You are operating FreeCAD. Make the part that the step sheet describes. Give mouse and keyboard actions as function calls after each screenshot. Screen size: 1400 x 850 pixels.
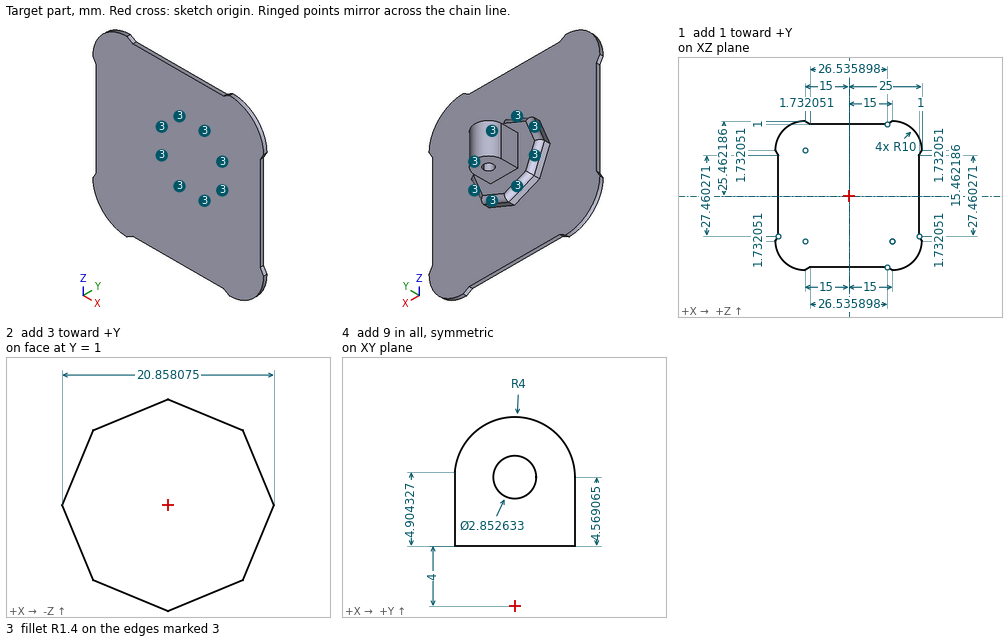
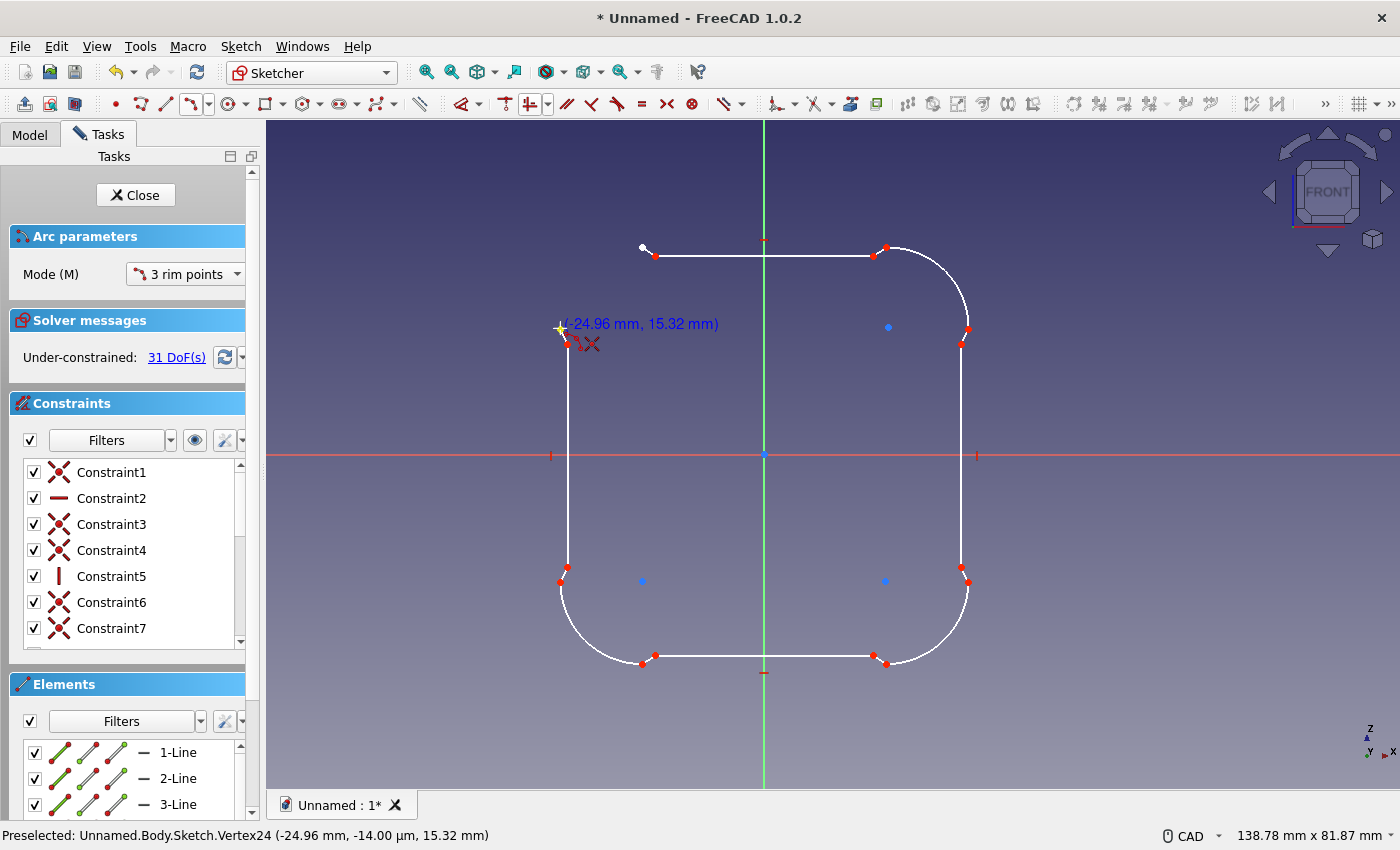
scroll(642, 247, up, 4)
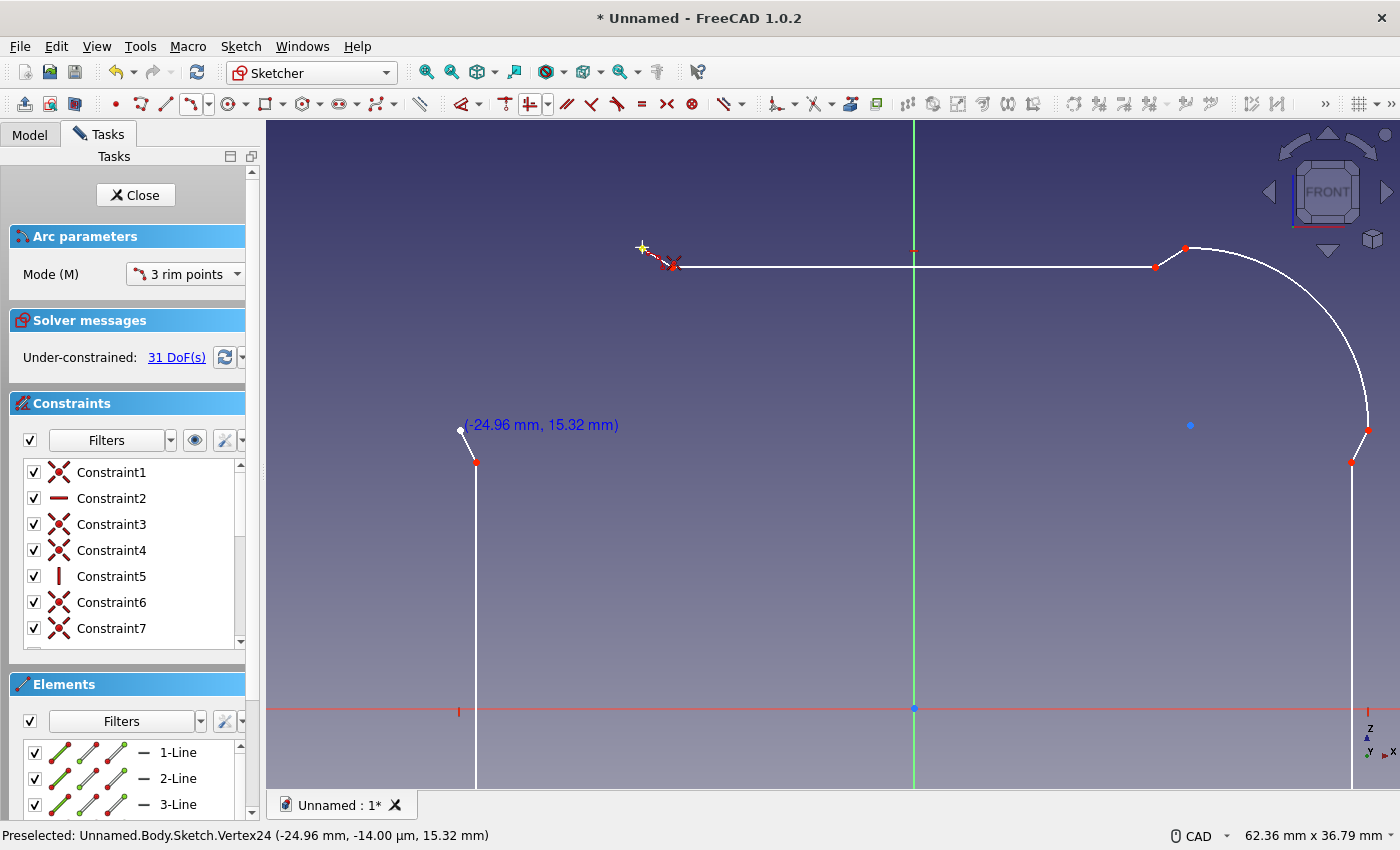
click(642, 248)
click(513, 299)
key(Escape)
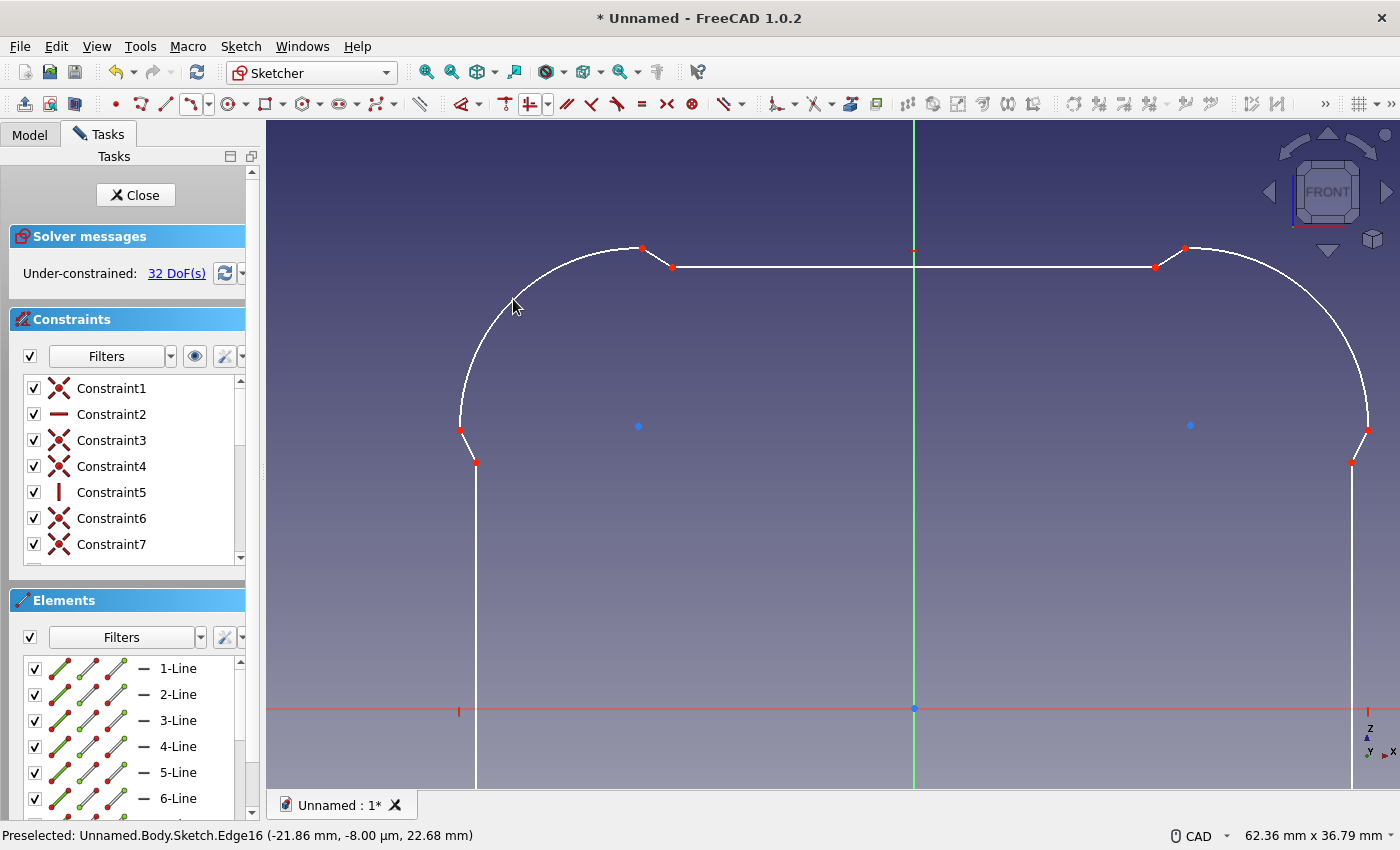
scroll(642, 247, down, 4)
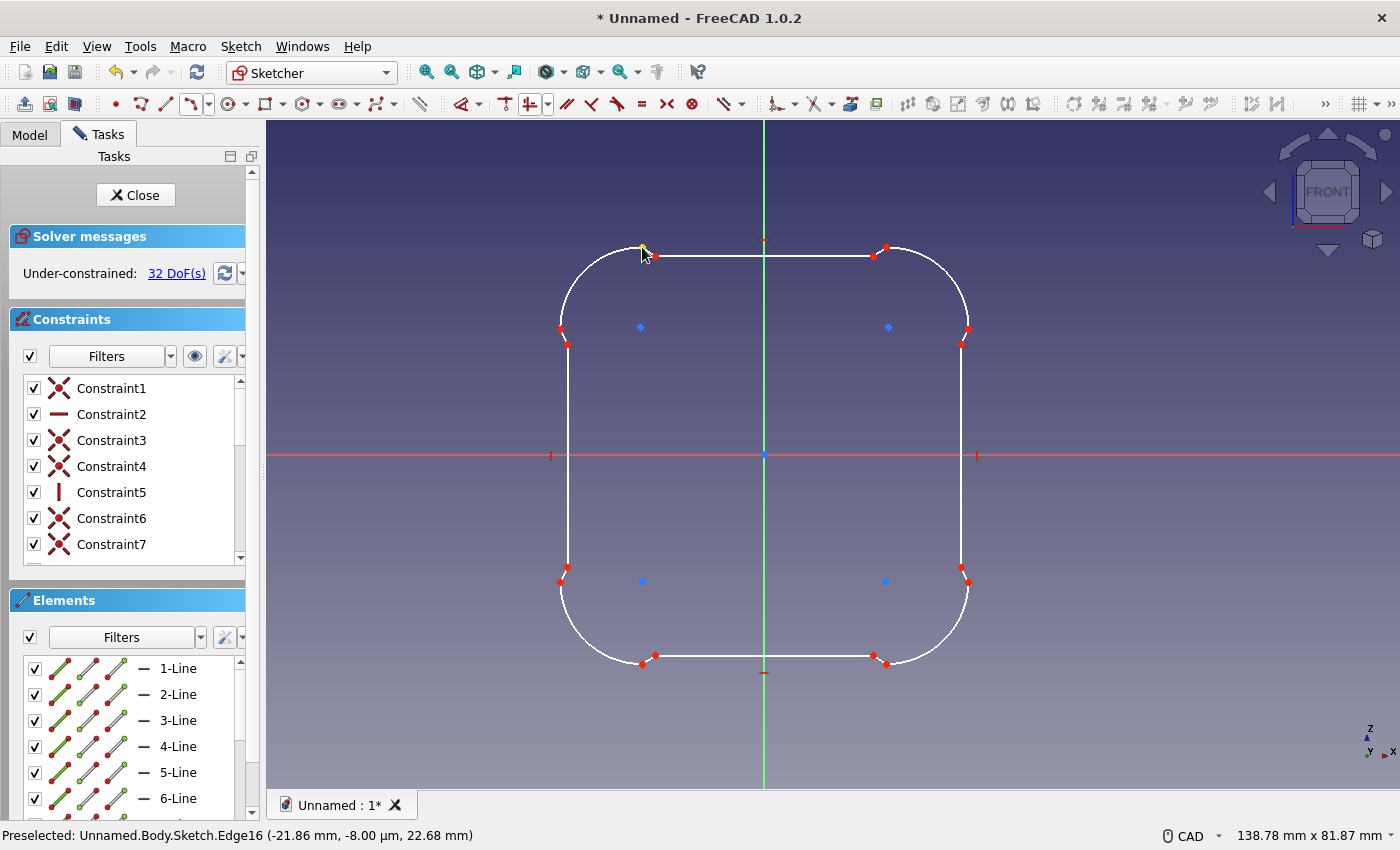
click(960, 292)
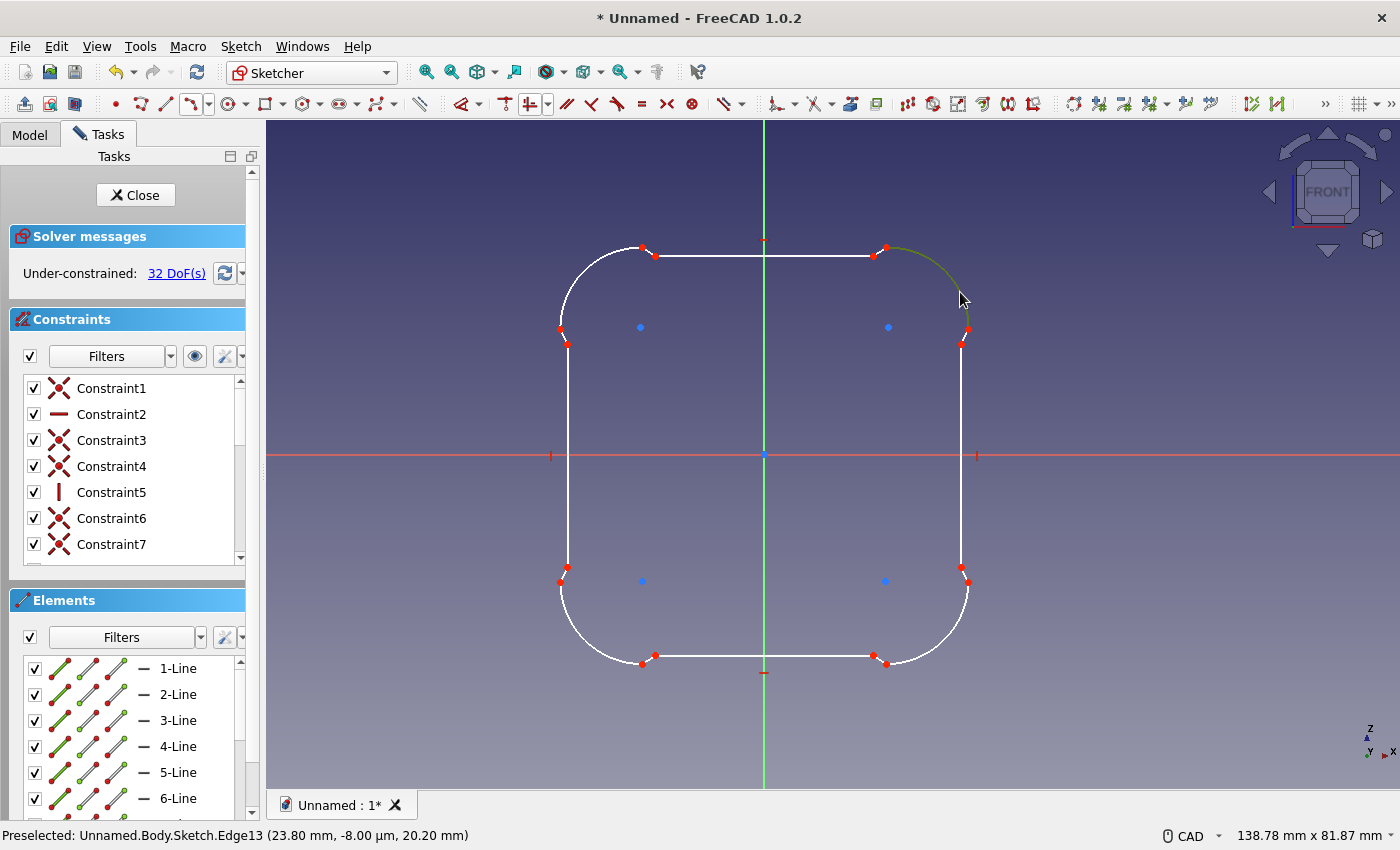
click(924, 655)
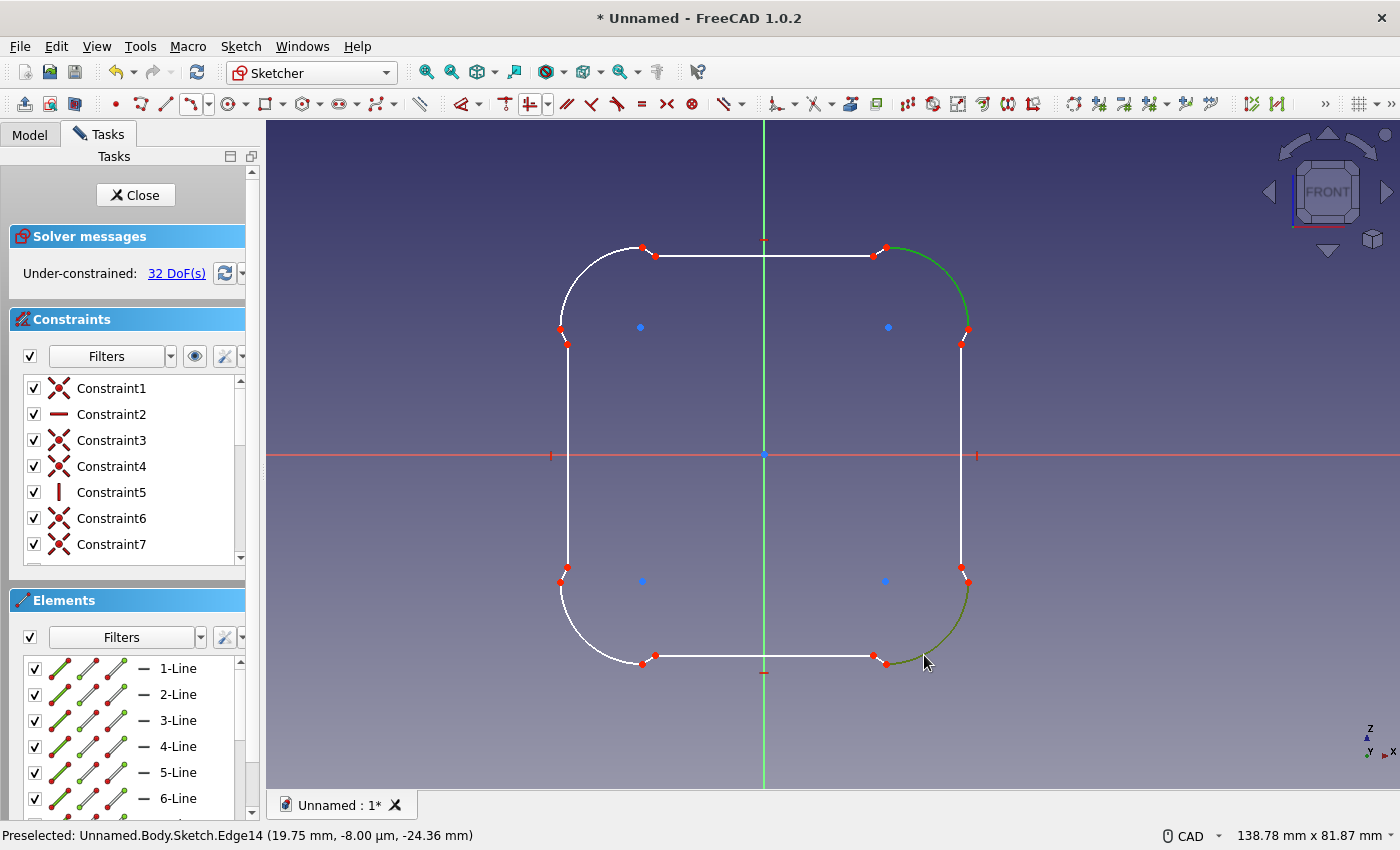
click(570, 619)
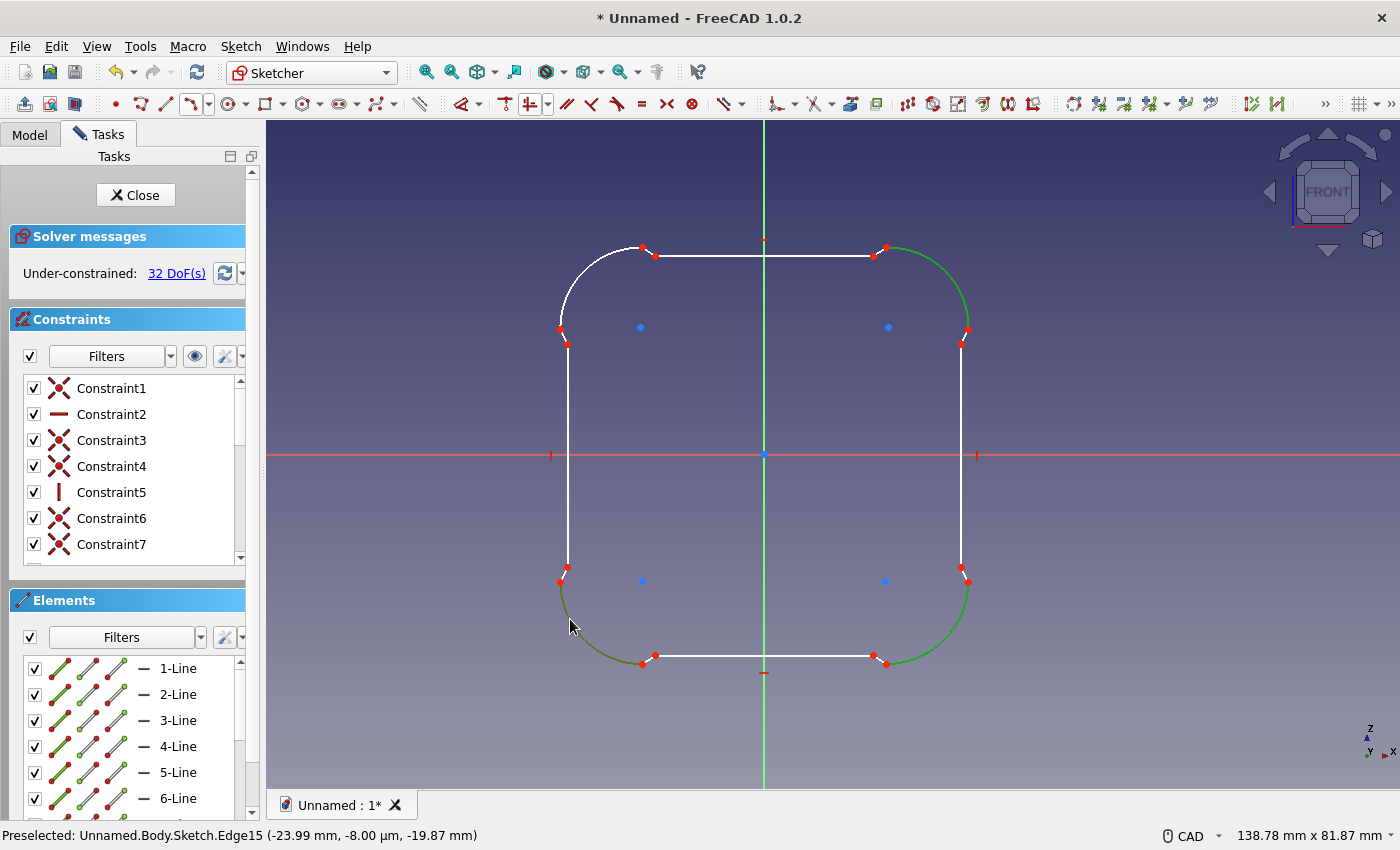
click(605, 256)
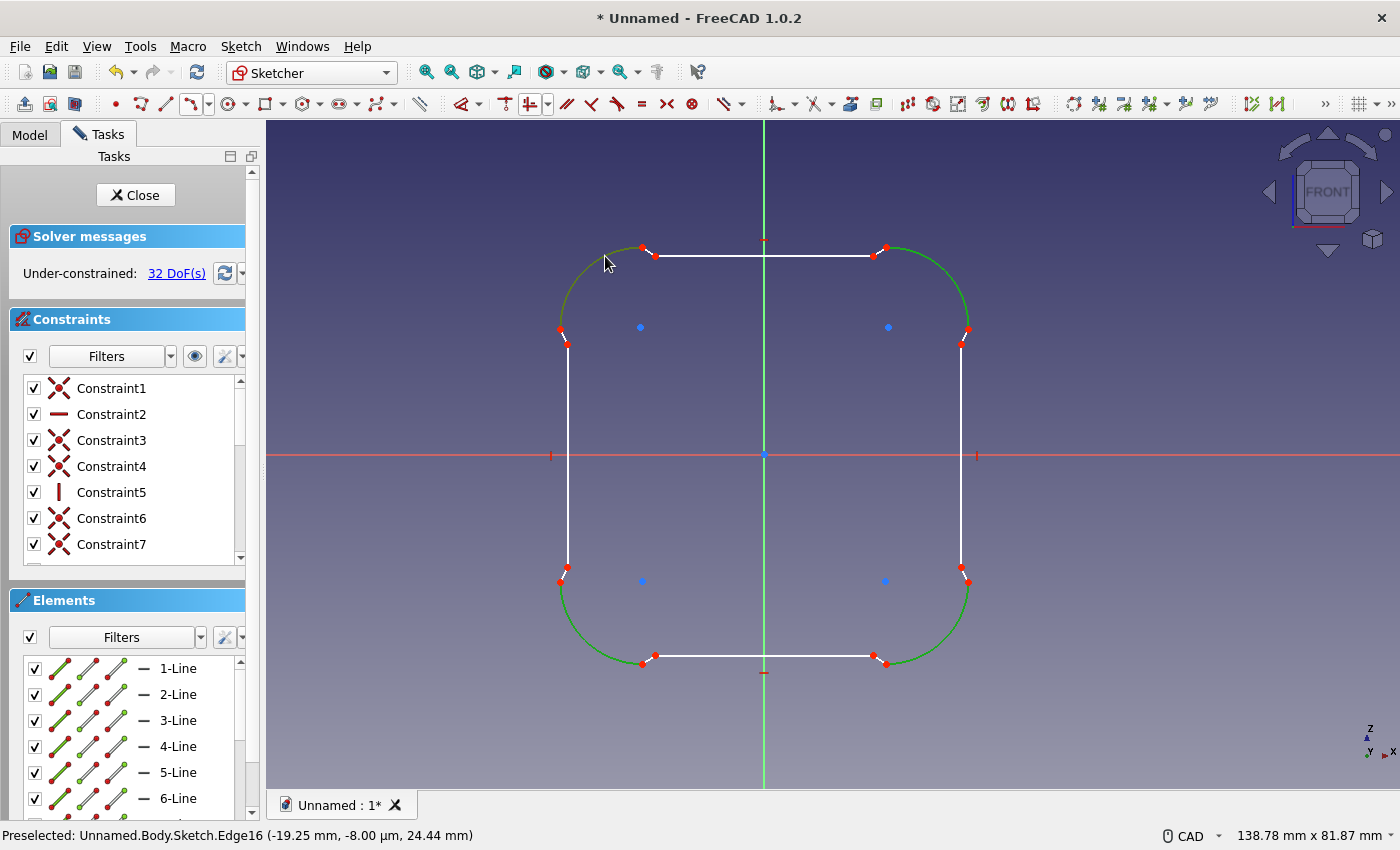
click(642, 104)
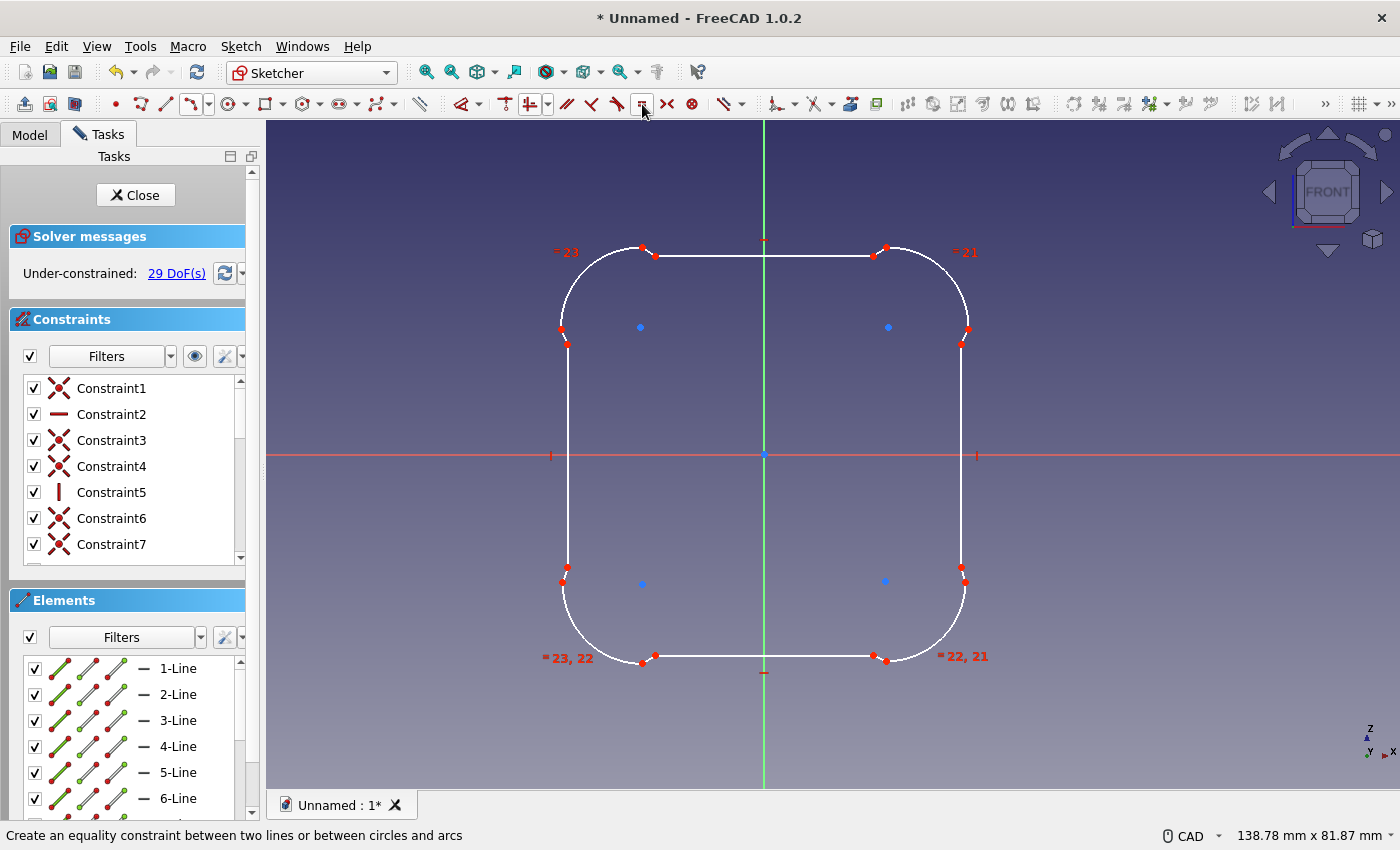
click(889, 327)